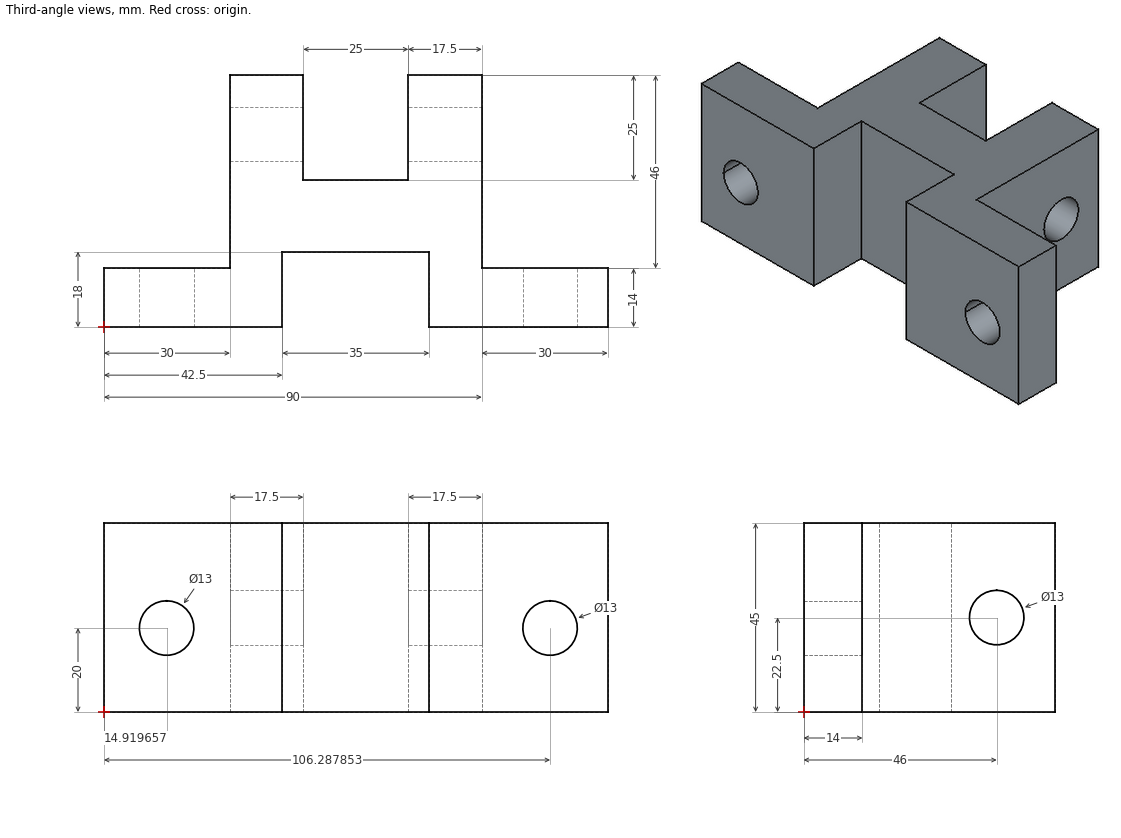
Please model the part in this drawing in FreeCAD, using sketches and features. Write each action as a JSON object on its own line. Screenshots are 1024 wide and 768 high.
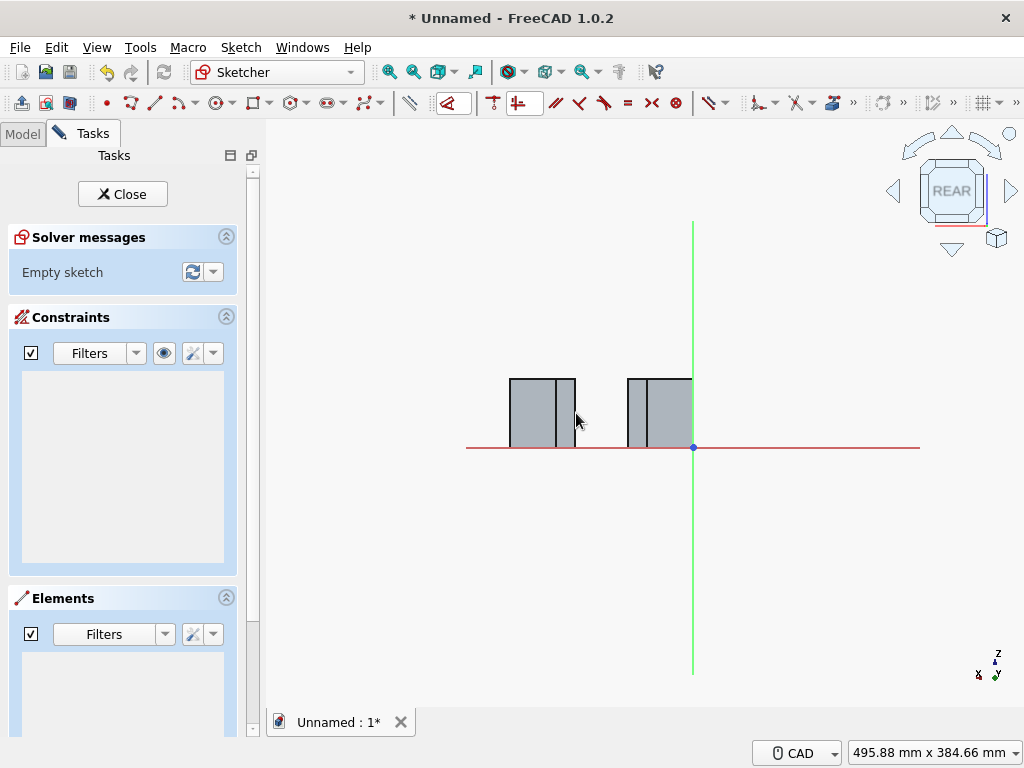
{"action": "scroll", "coordinate": [690, 429], "scroll_direction": "up", "scroll_amount": 11}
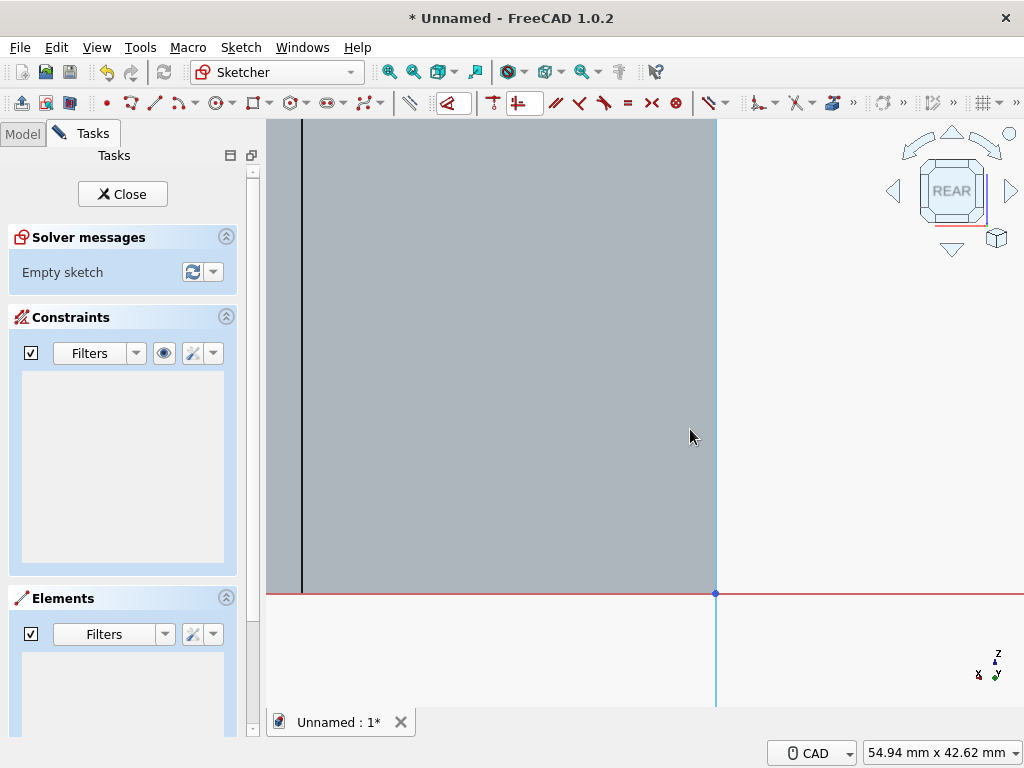
{"action": "left_click", "coordinate": [216, 104]}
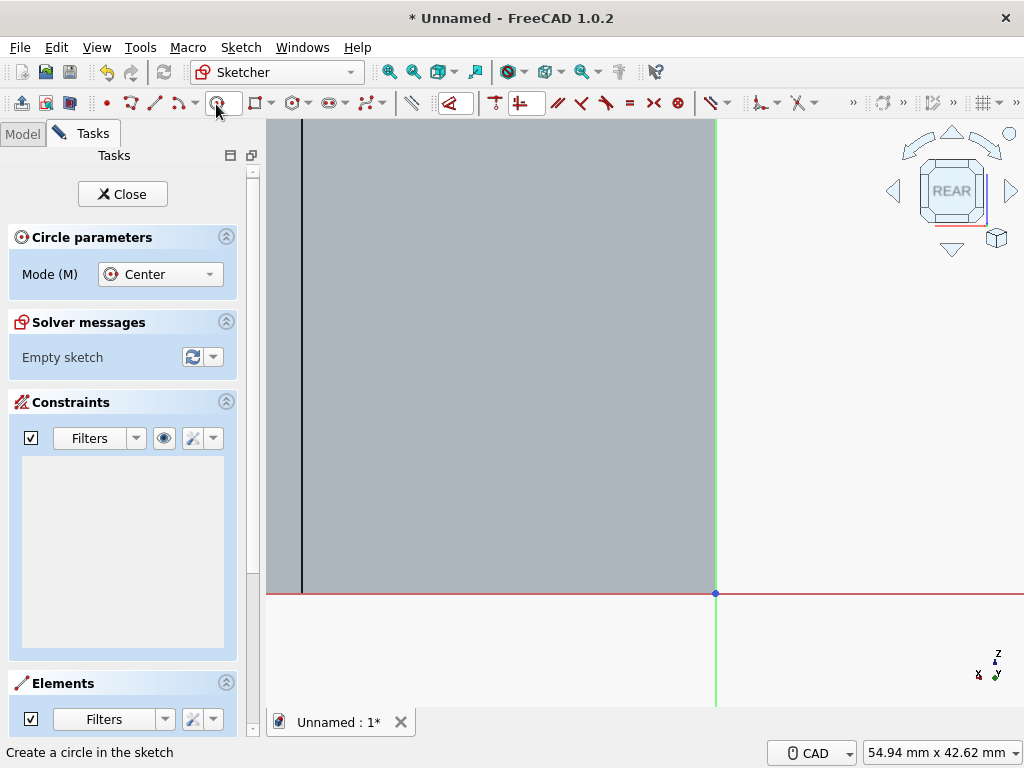
{"action": "left_click", "coordinate": [510, 318]}
{"action": "mouse_move", "coordinate": [573, 254]}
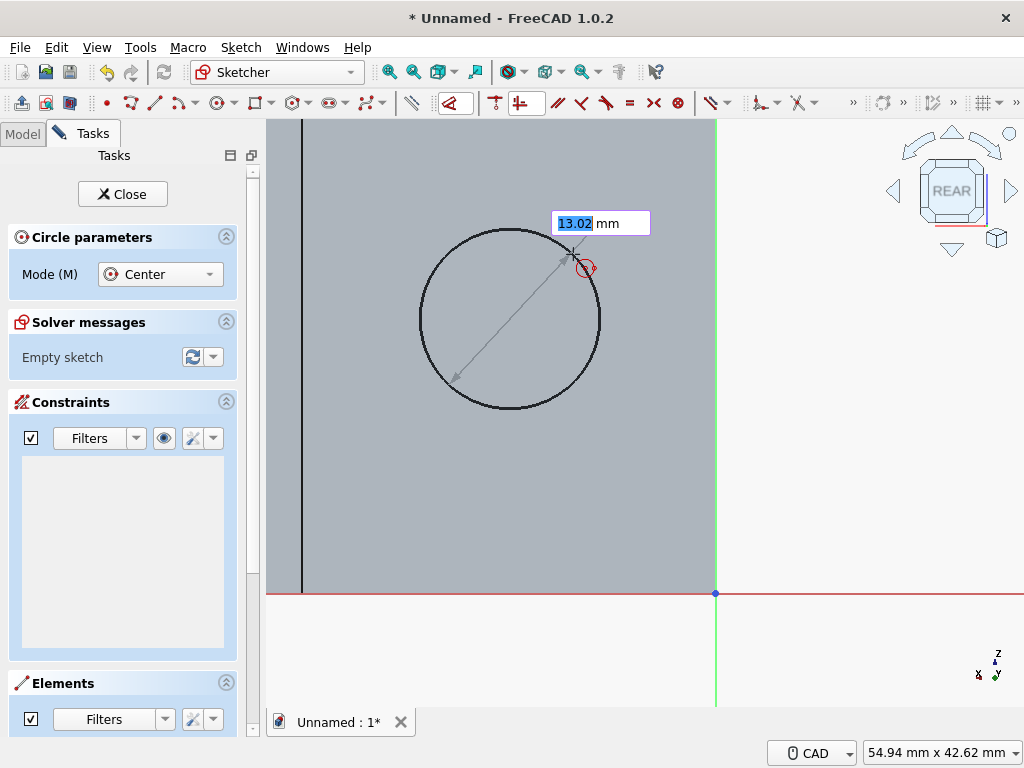
{"action": "type", "text": "13"}
{"action": "key", "text": "Return"}
{"action": "key", "text": "Escape"}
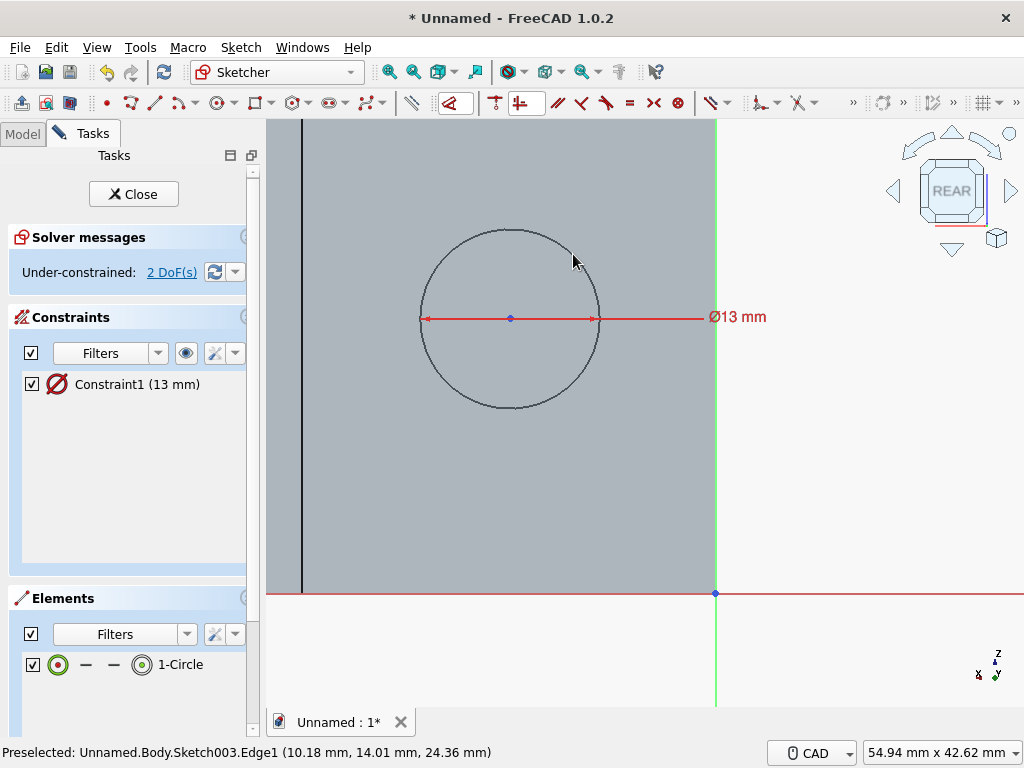
{"action": "left_click", "coordinate": [510, 319]}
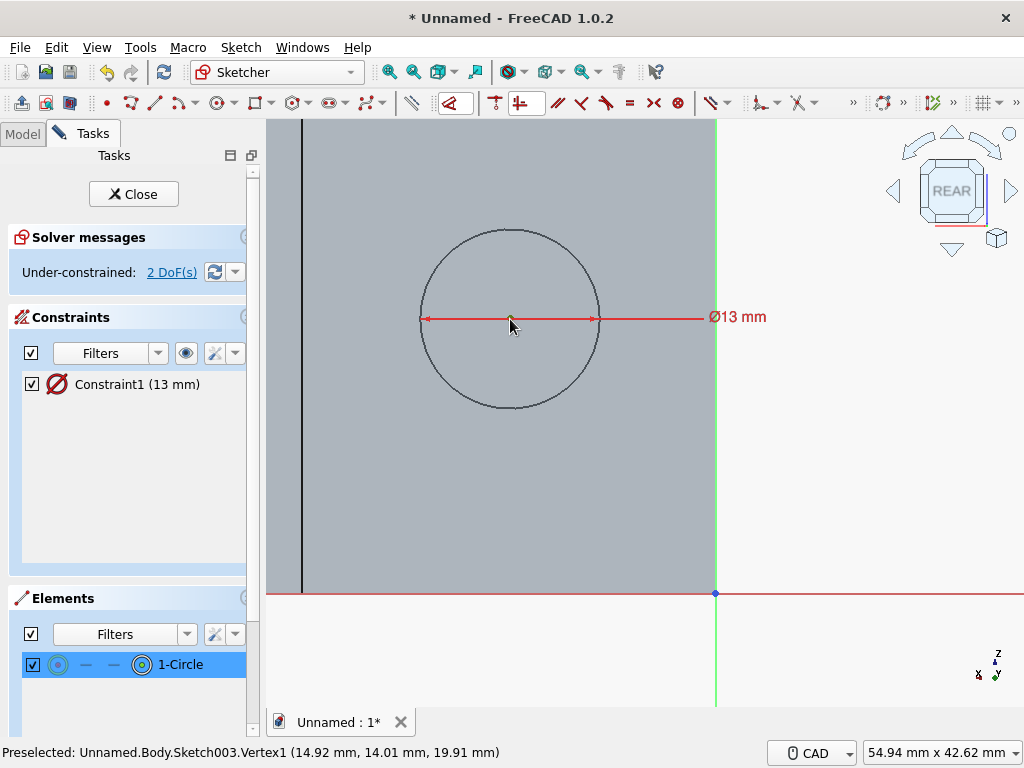
{"action": "key", "text": "i"}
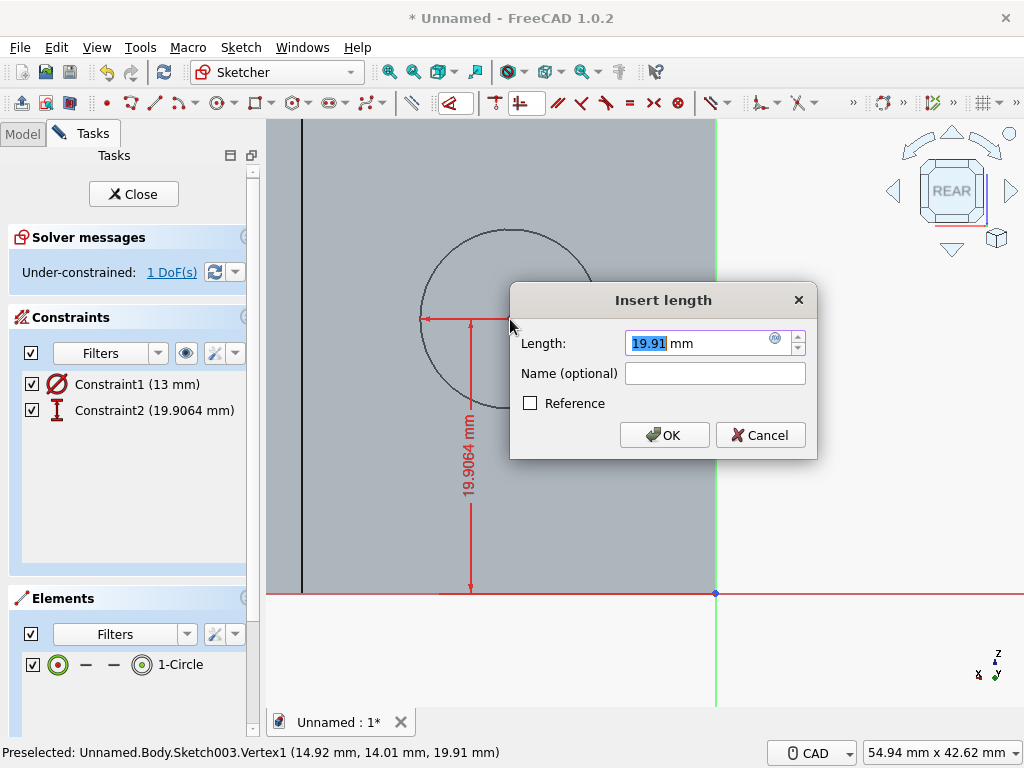
{"action": "type", "text": "20"}
{"action": "key", "text": "Return"}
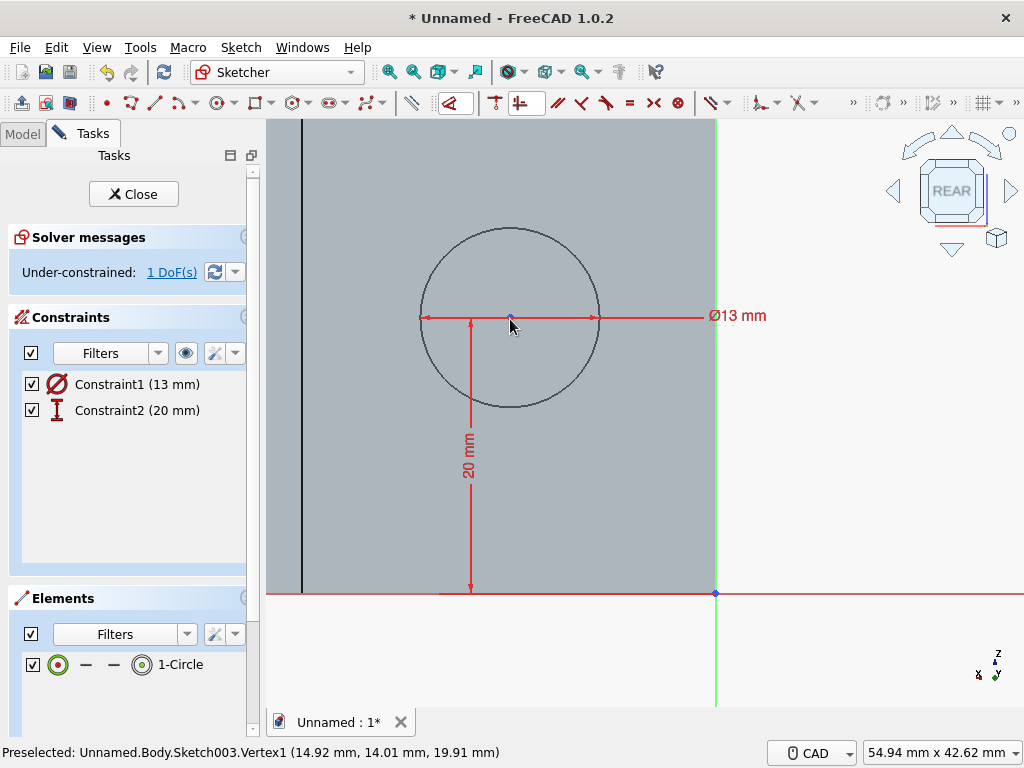
{"action": "left_click", "coordinate": [510, 318]}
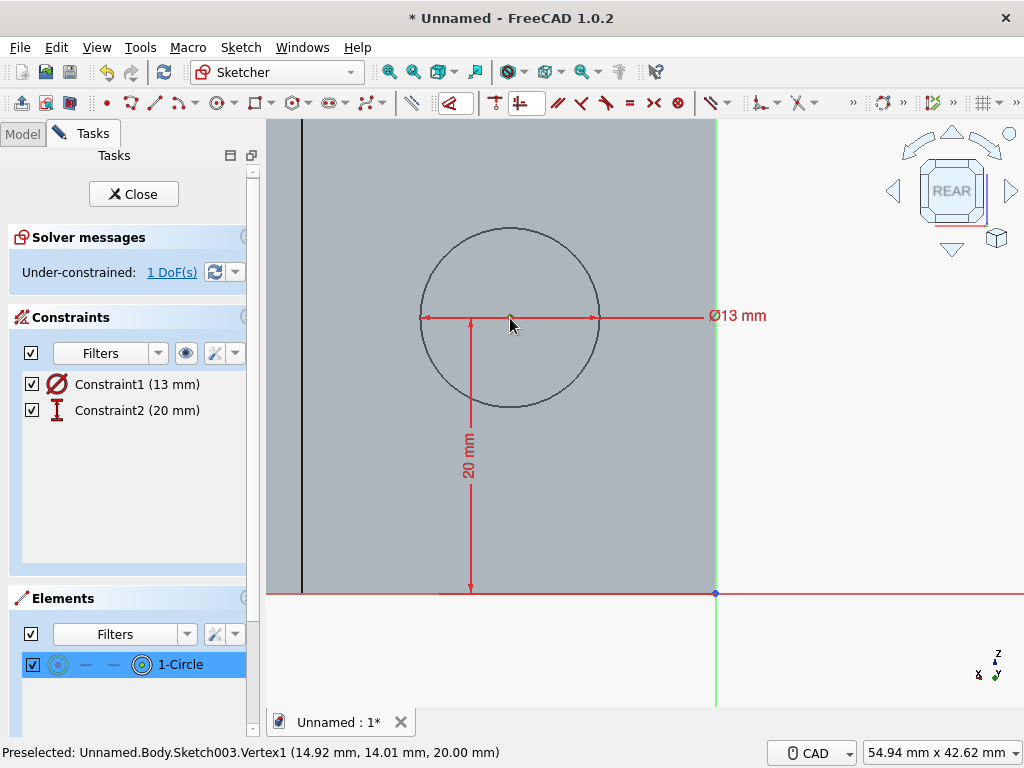
{"action": "left_click", "coordinate": [468, 104]}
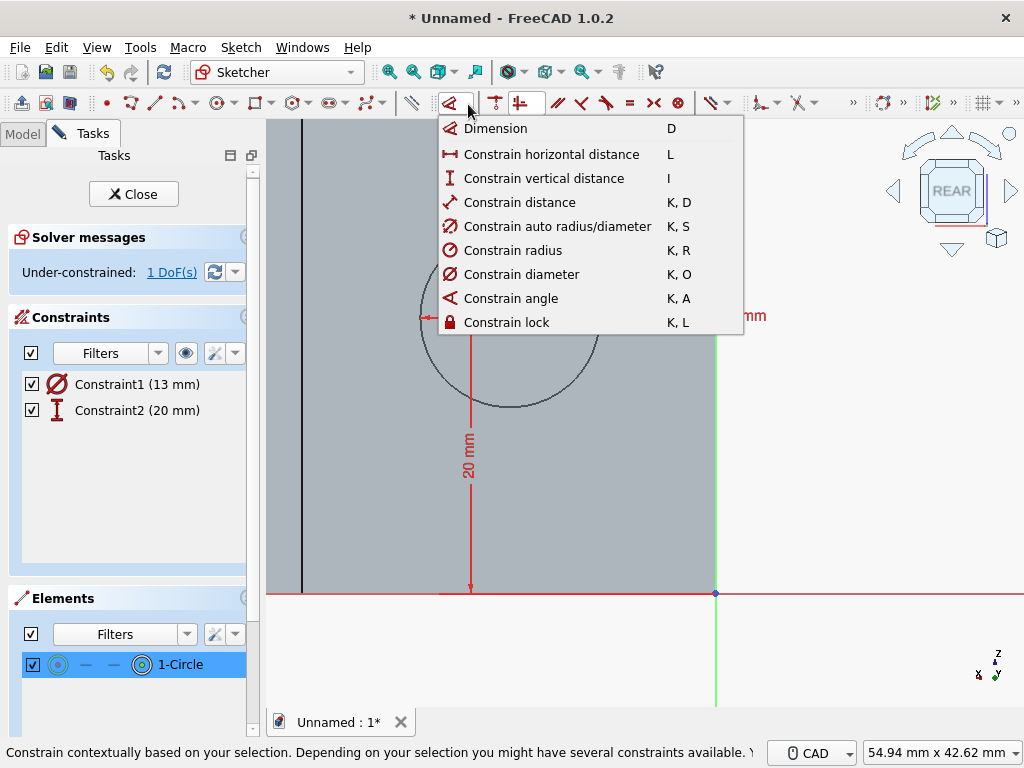
{"action": "left_click", "coordinate": [591, 154]}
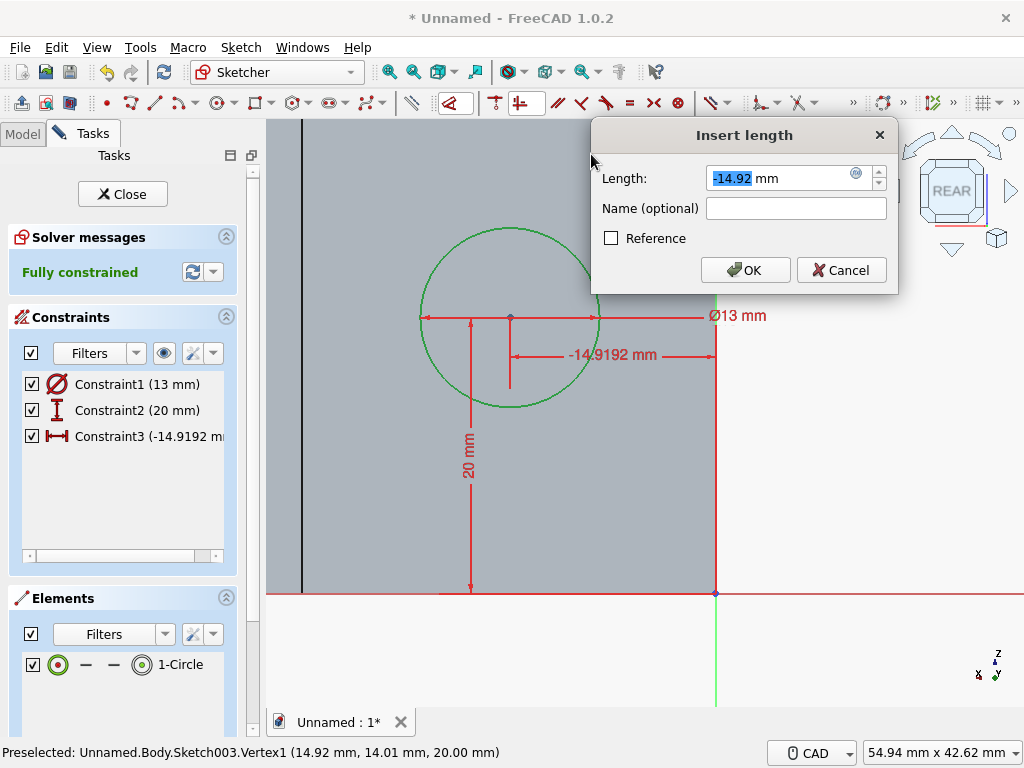
{"action": "type", "text": "-14.919657"}
{"action": "key", "text": "Return"}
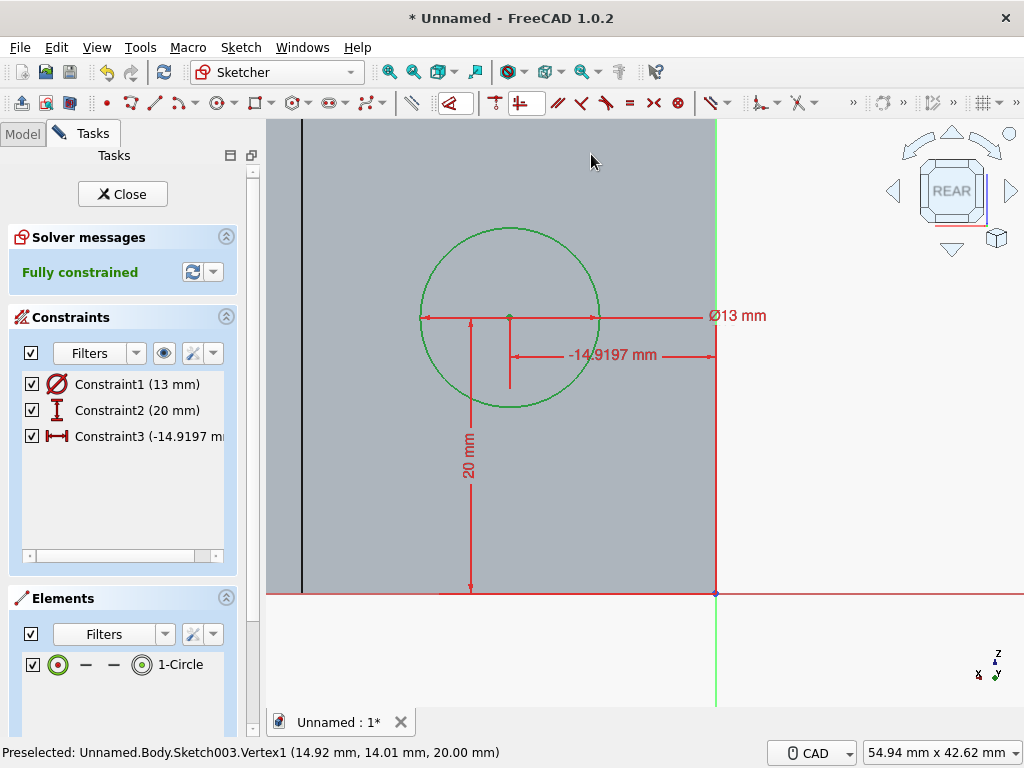
{"action": "left_click", "coordinate": [123, 194]}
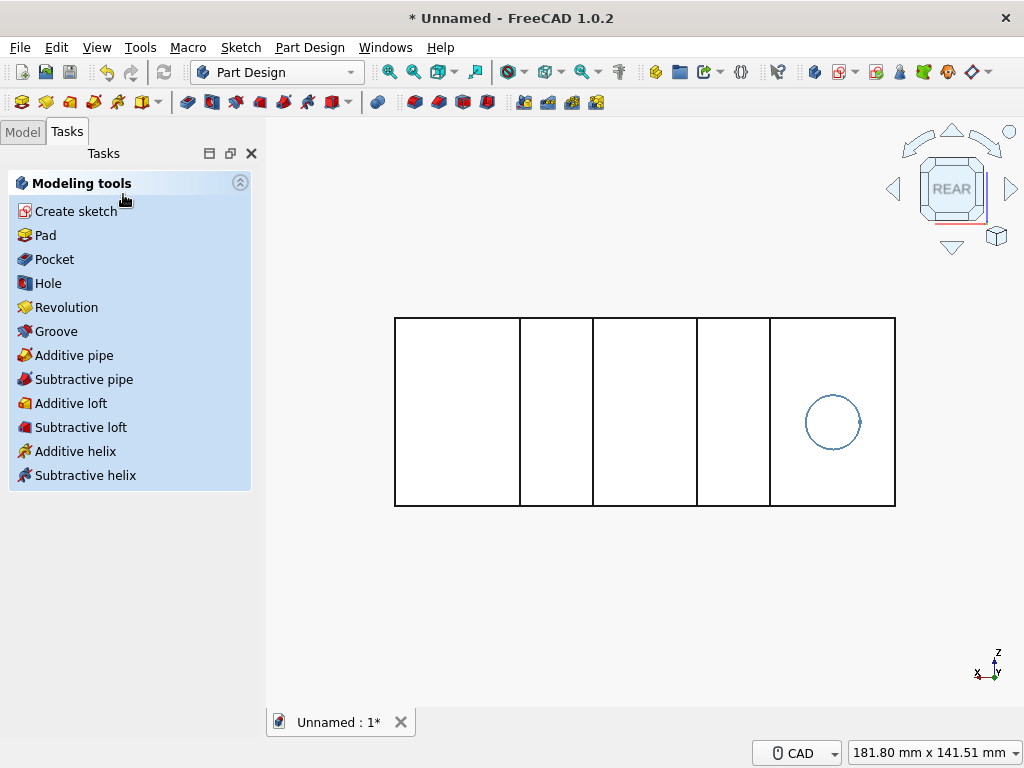
{"action": "left_click", "coordinate": [188, 102]}